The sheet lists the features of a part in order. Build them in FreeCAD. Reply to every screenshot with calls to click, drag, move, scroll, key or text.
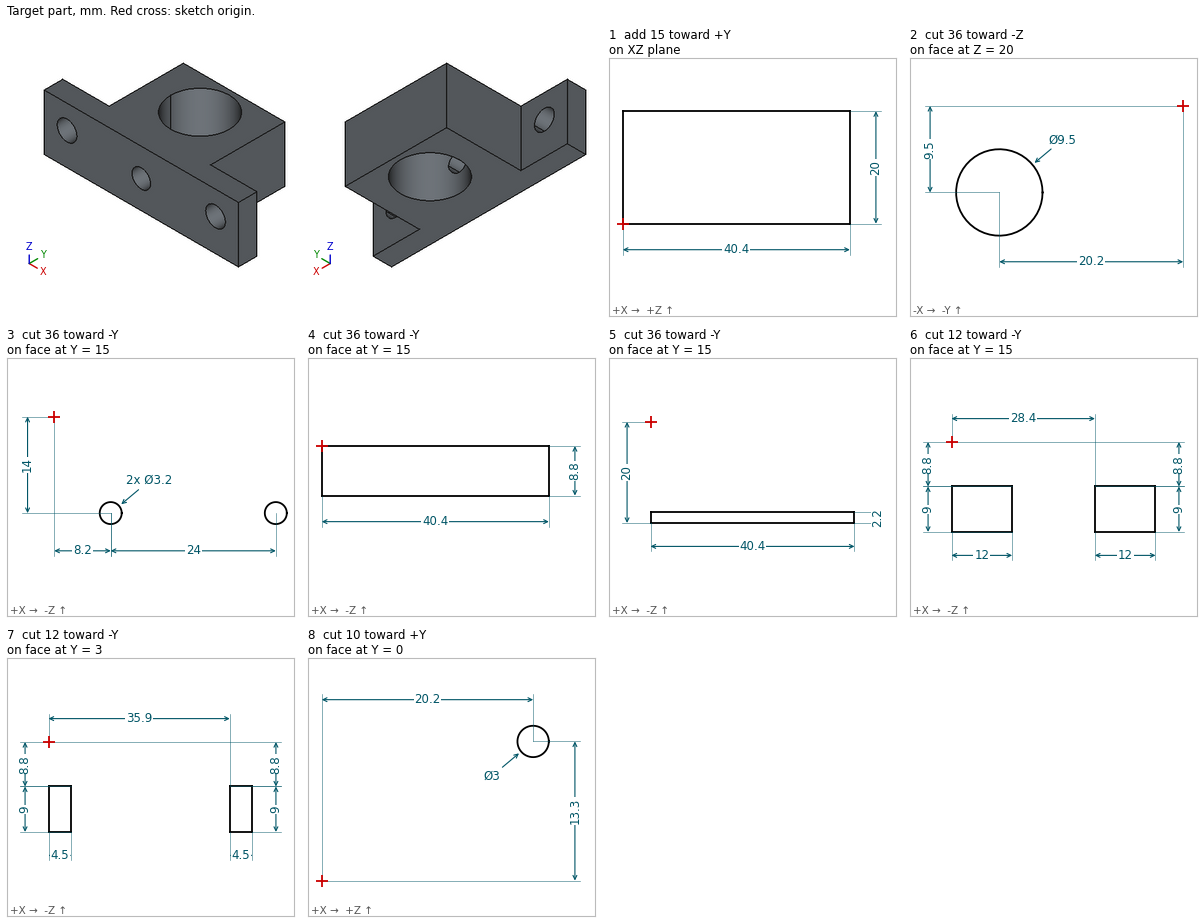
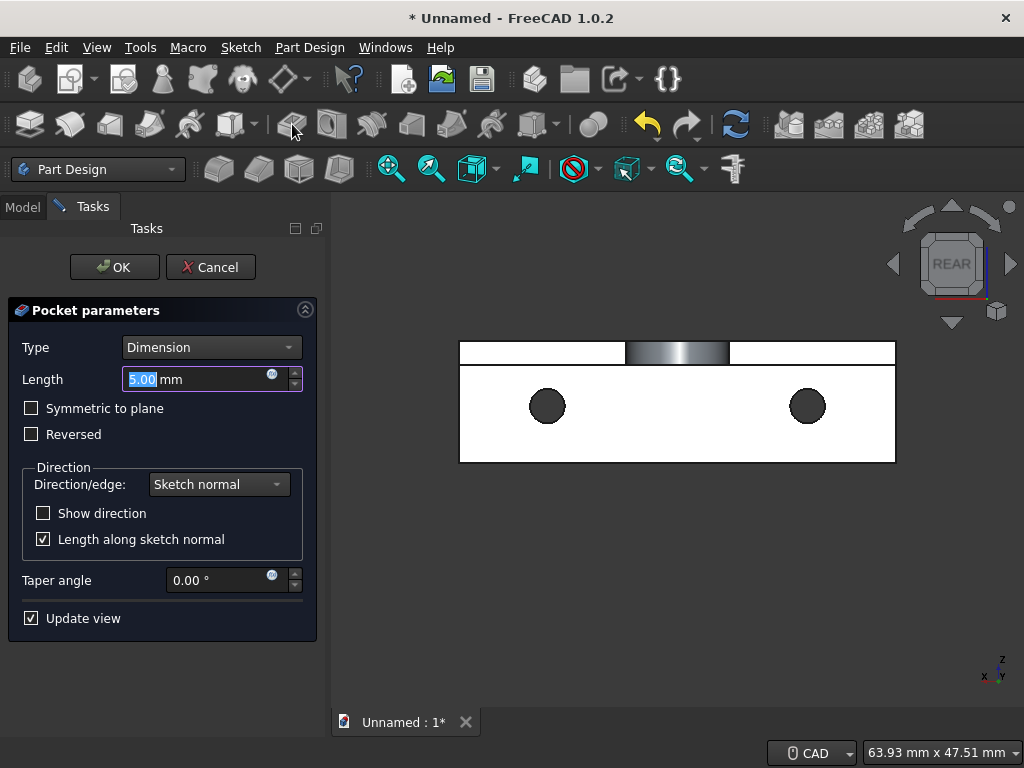
text(36)
key(Tab)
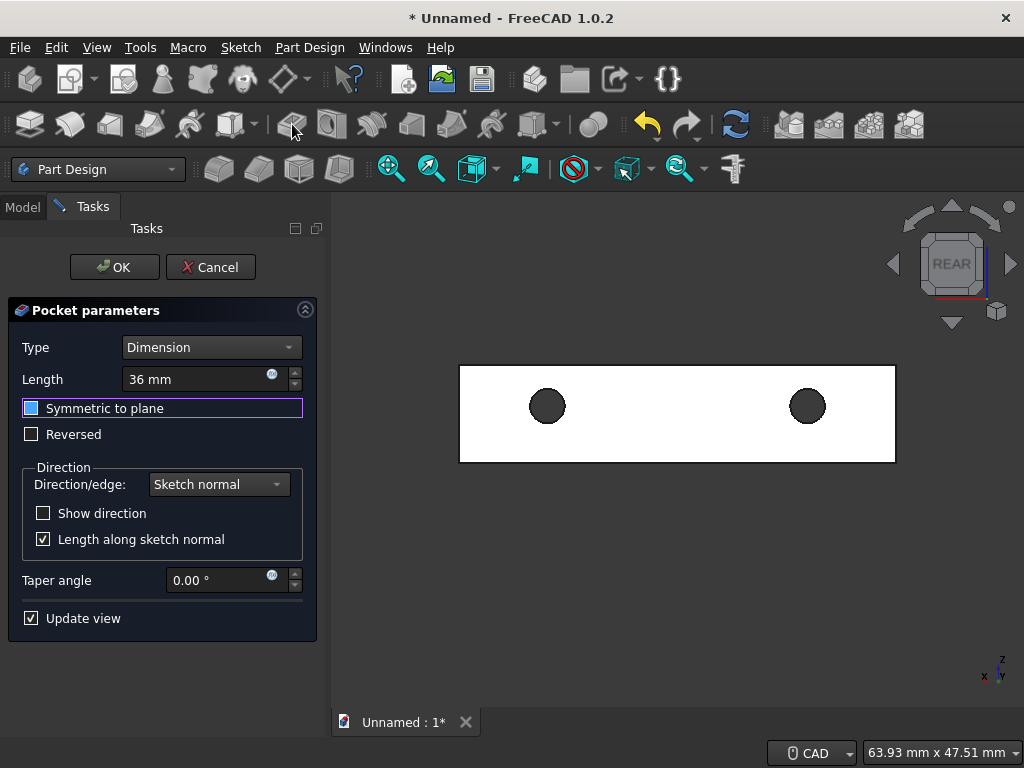
click(115, 267)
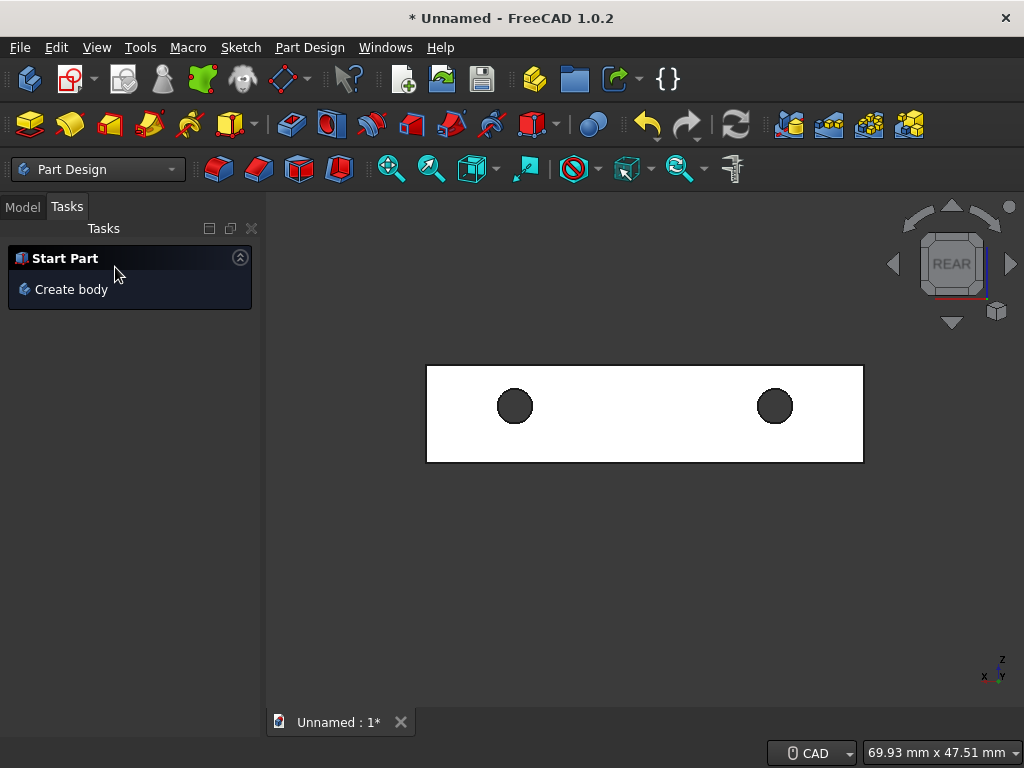
click(582, 413)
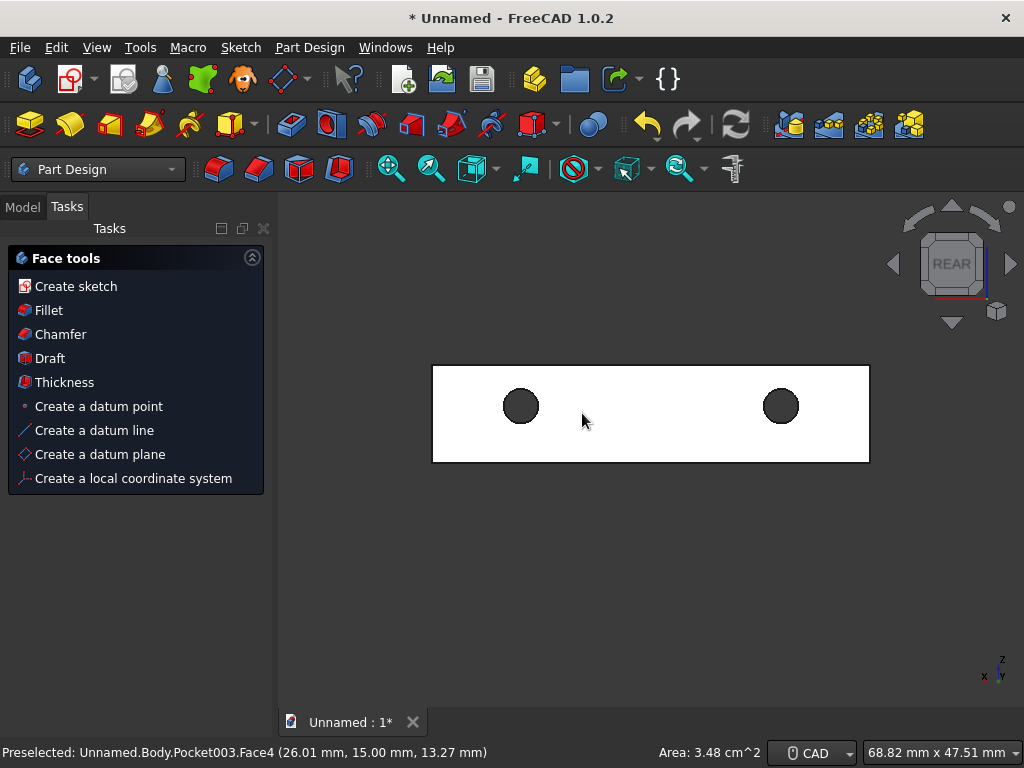
click(70, 80)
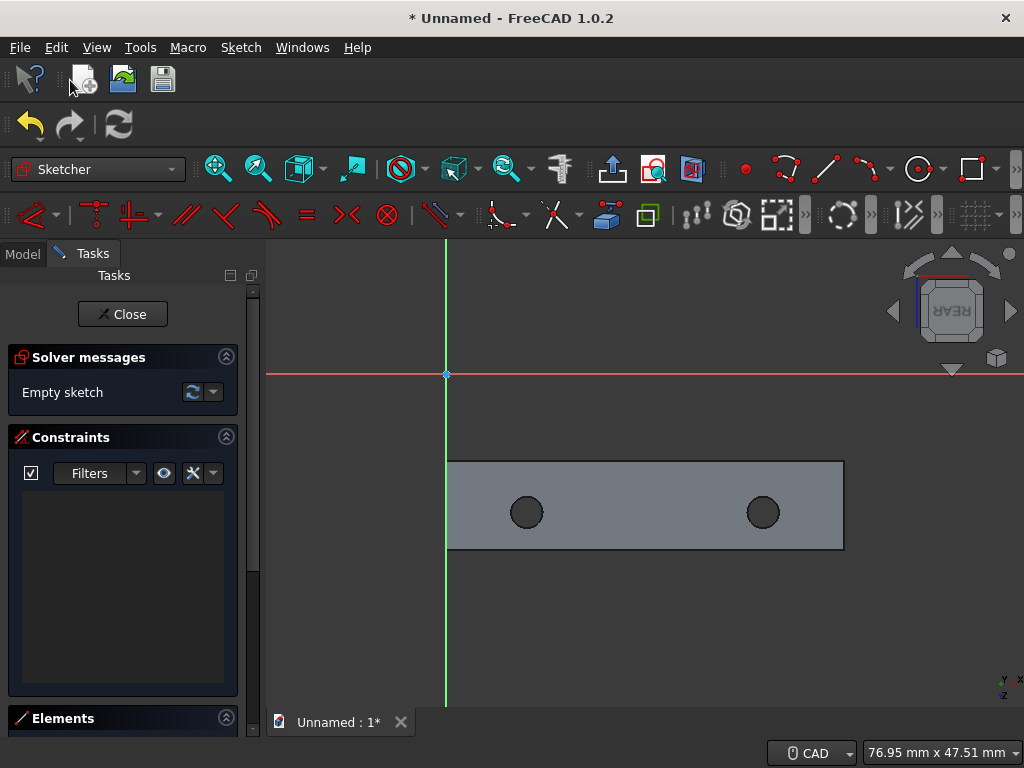
scroll(294, 522, down, 1)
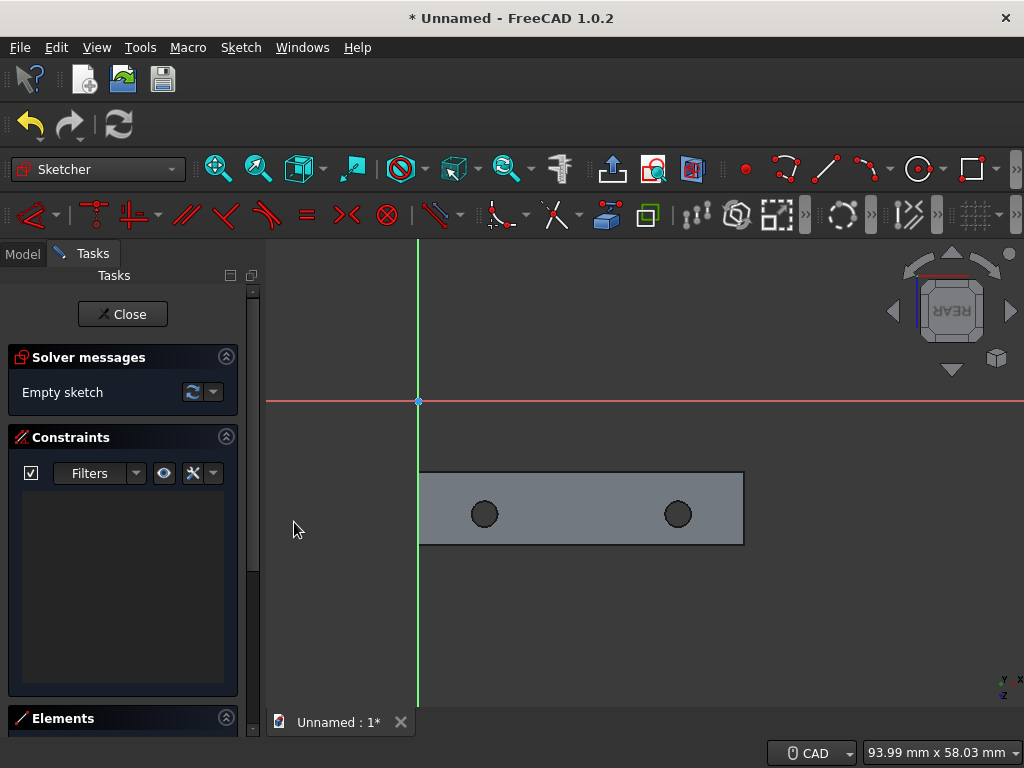
click(972, 170)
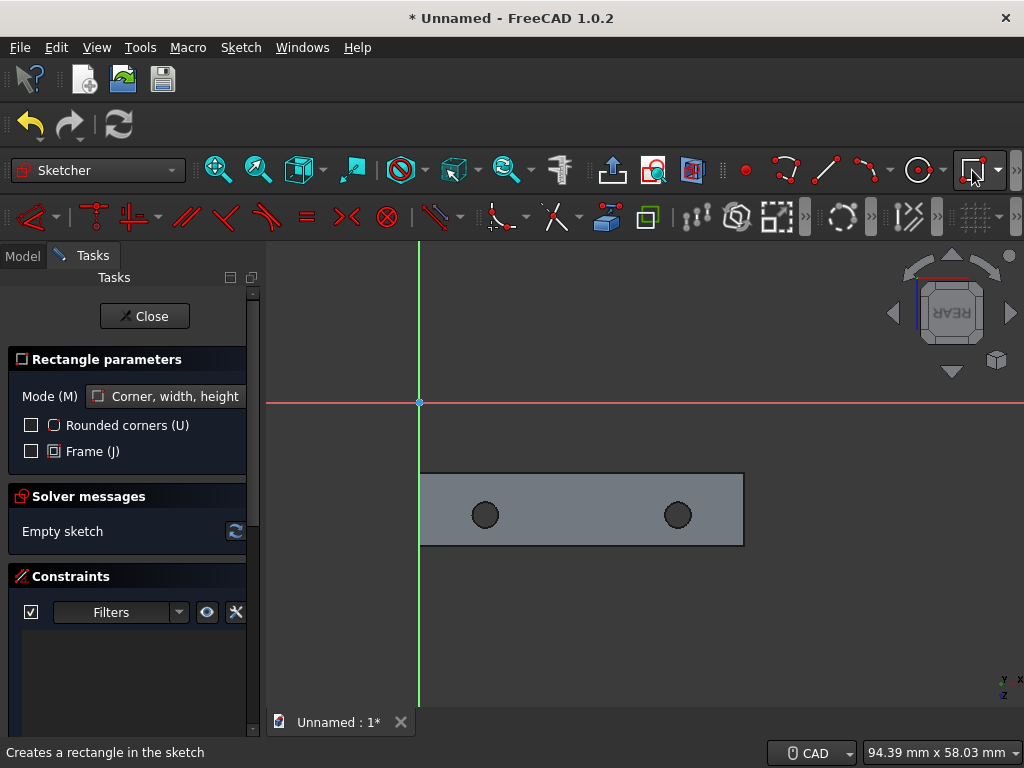
click(419, 473)
move(516, 546)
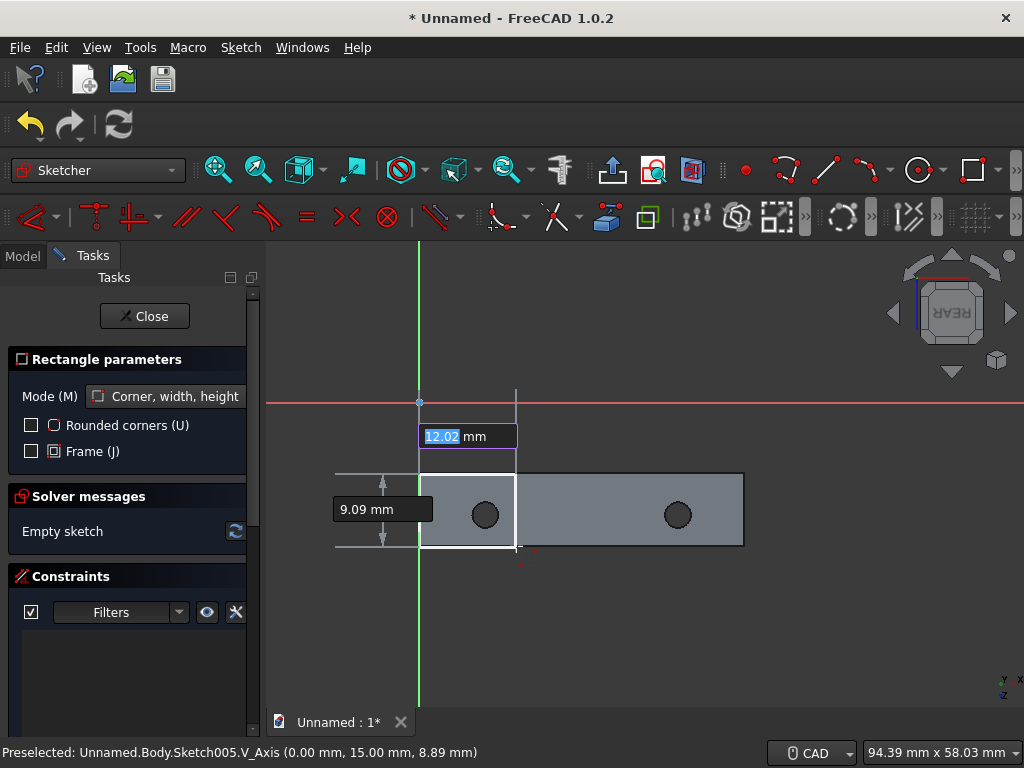
text(12)
key(Tab)
text(9)
key(Return)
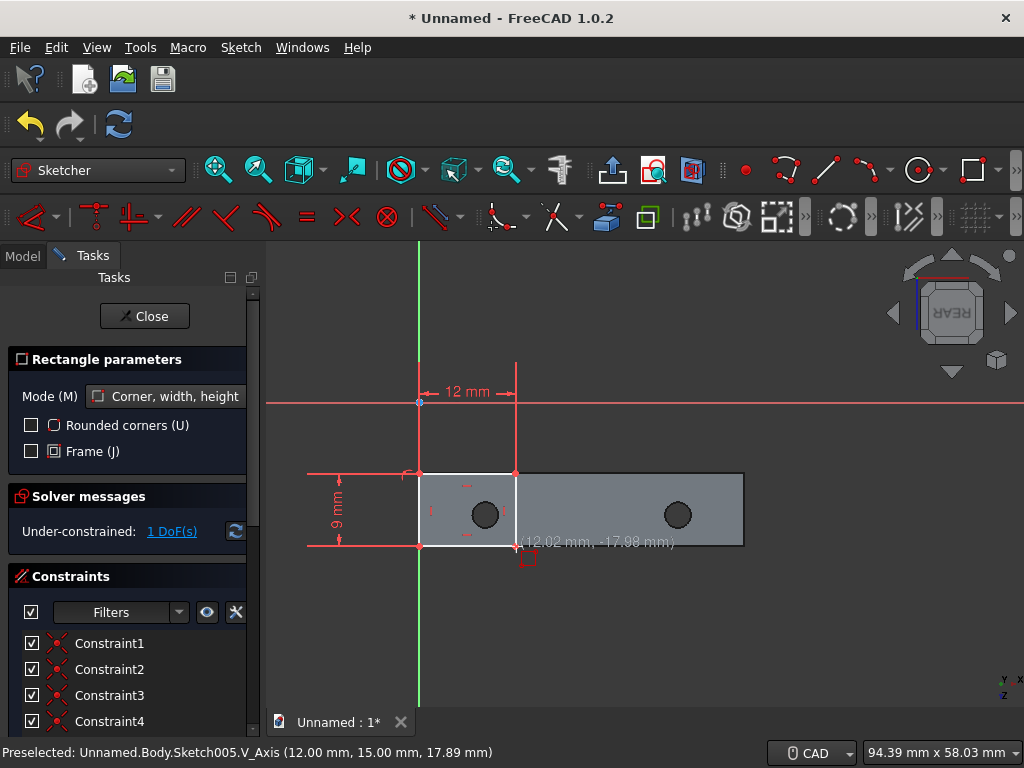
click(648, 473)
move(744, 546)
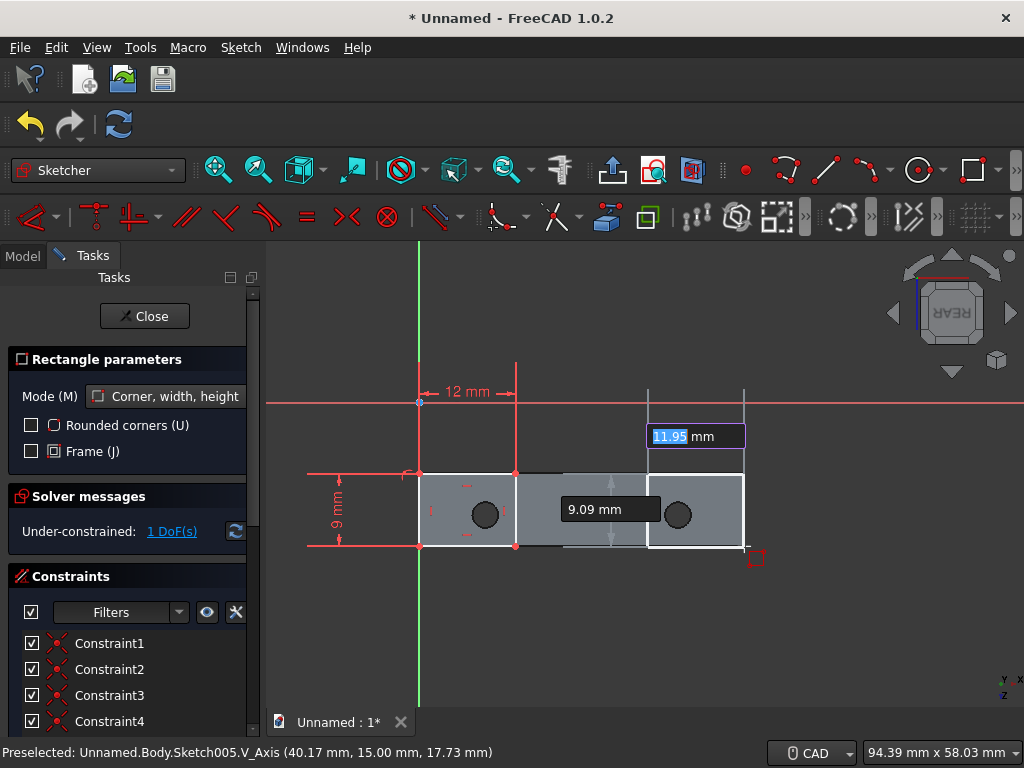
text(12)
key(Tab)
text(9)
key(Return)
key(Escape)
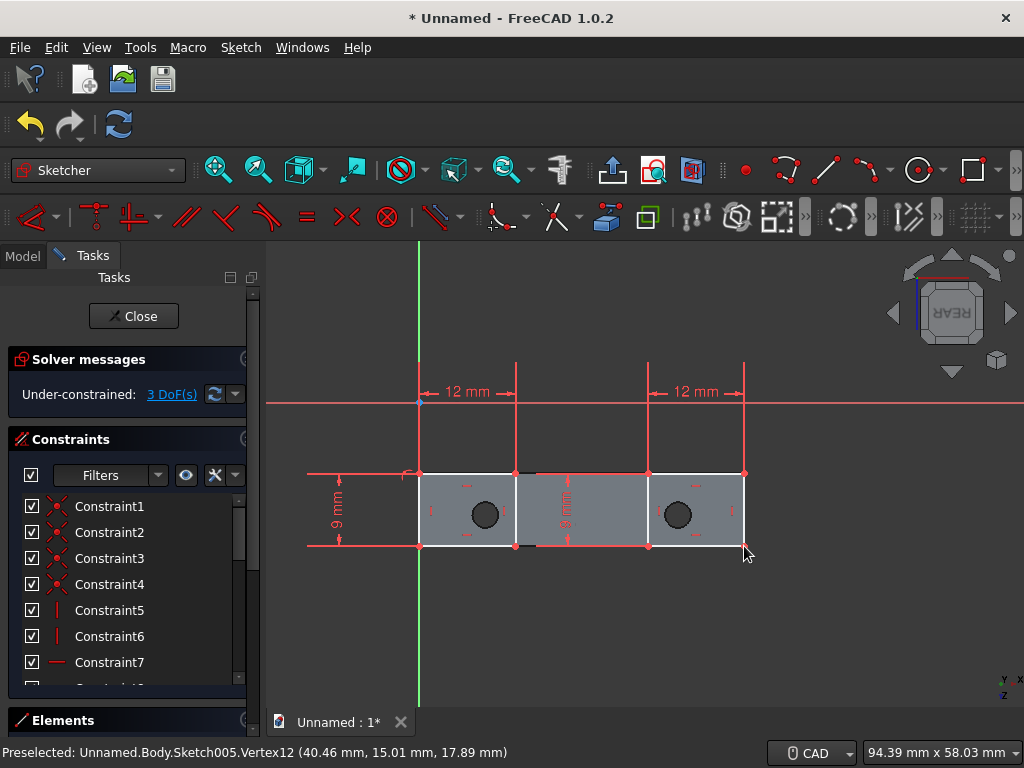
click(419, 474)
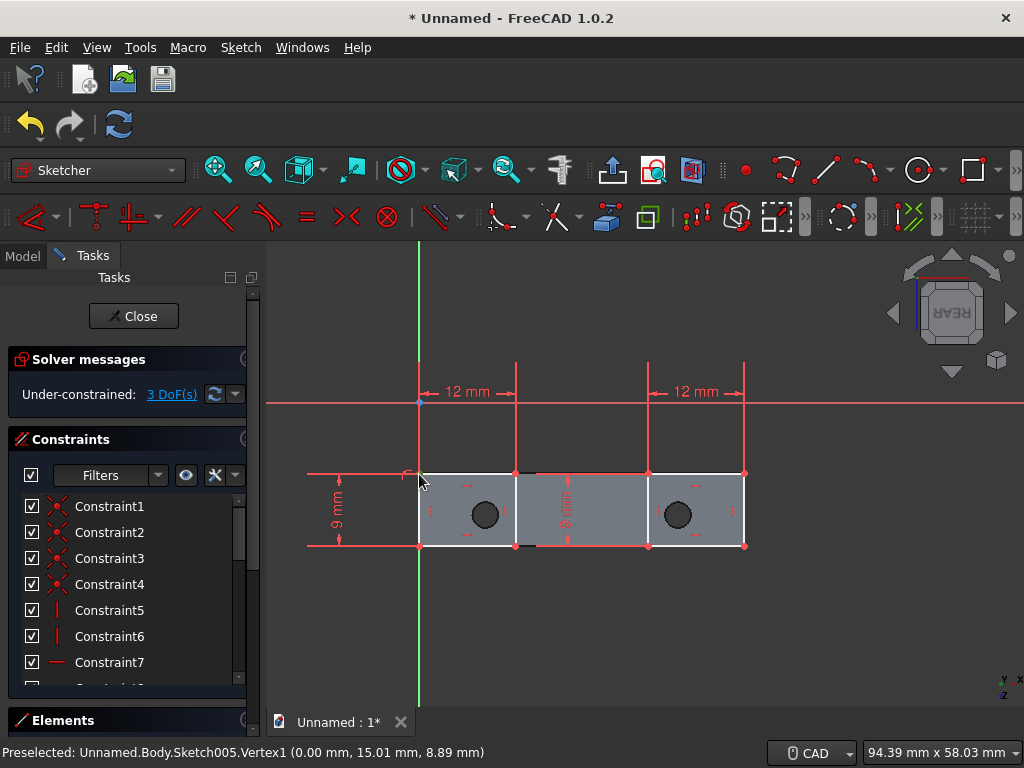
key(i)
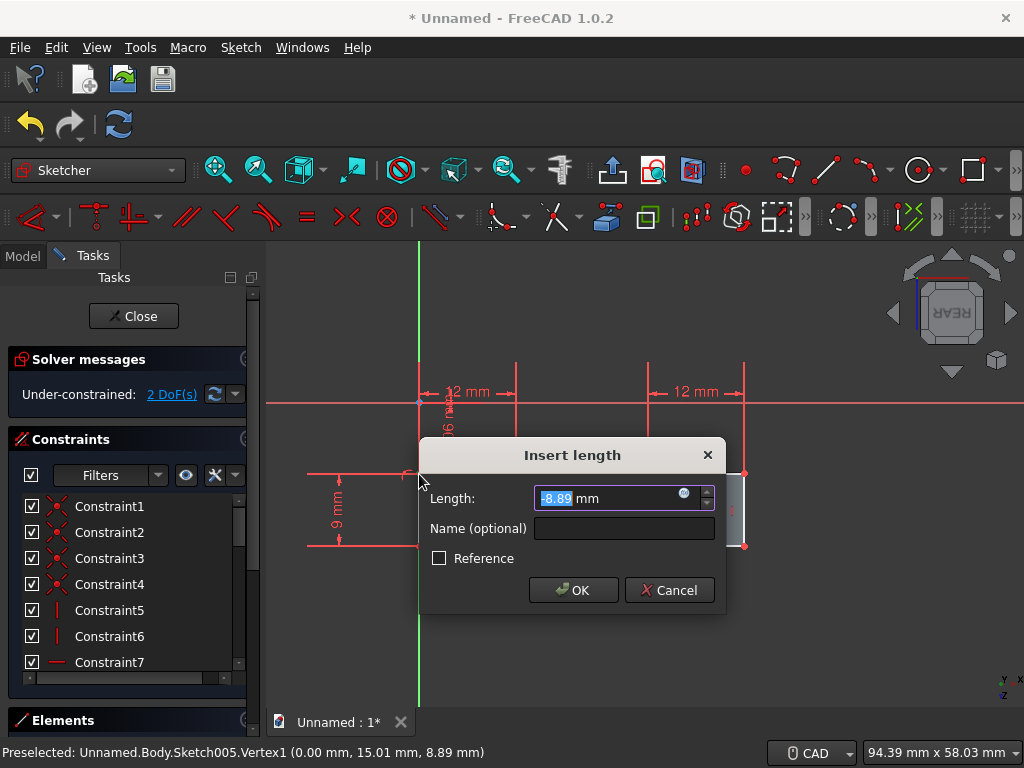
text(-8.8)
key(Return)